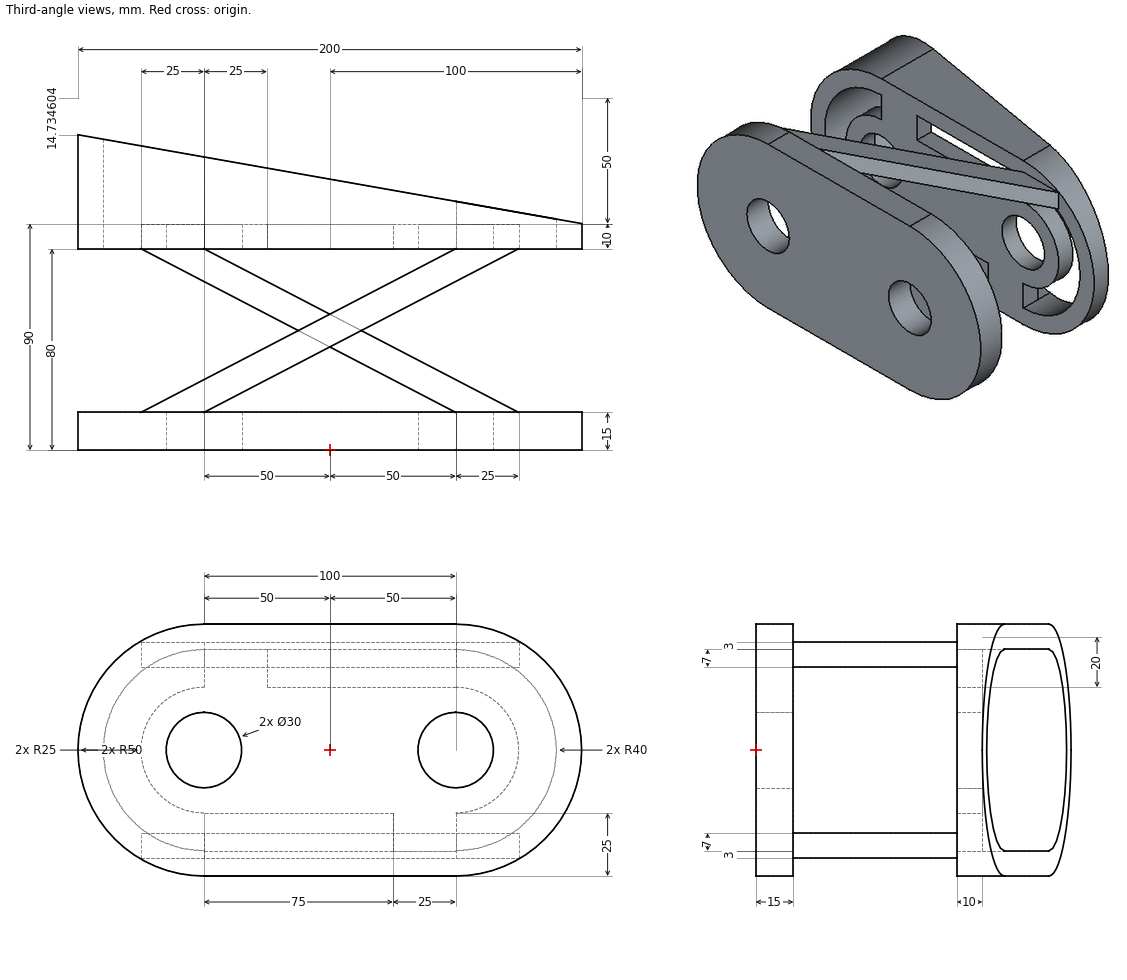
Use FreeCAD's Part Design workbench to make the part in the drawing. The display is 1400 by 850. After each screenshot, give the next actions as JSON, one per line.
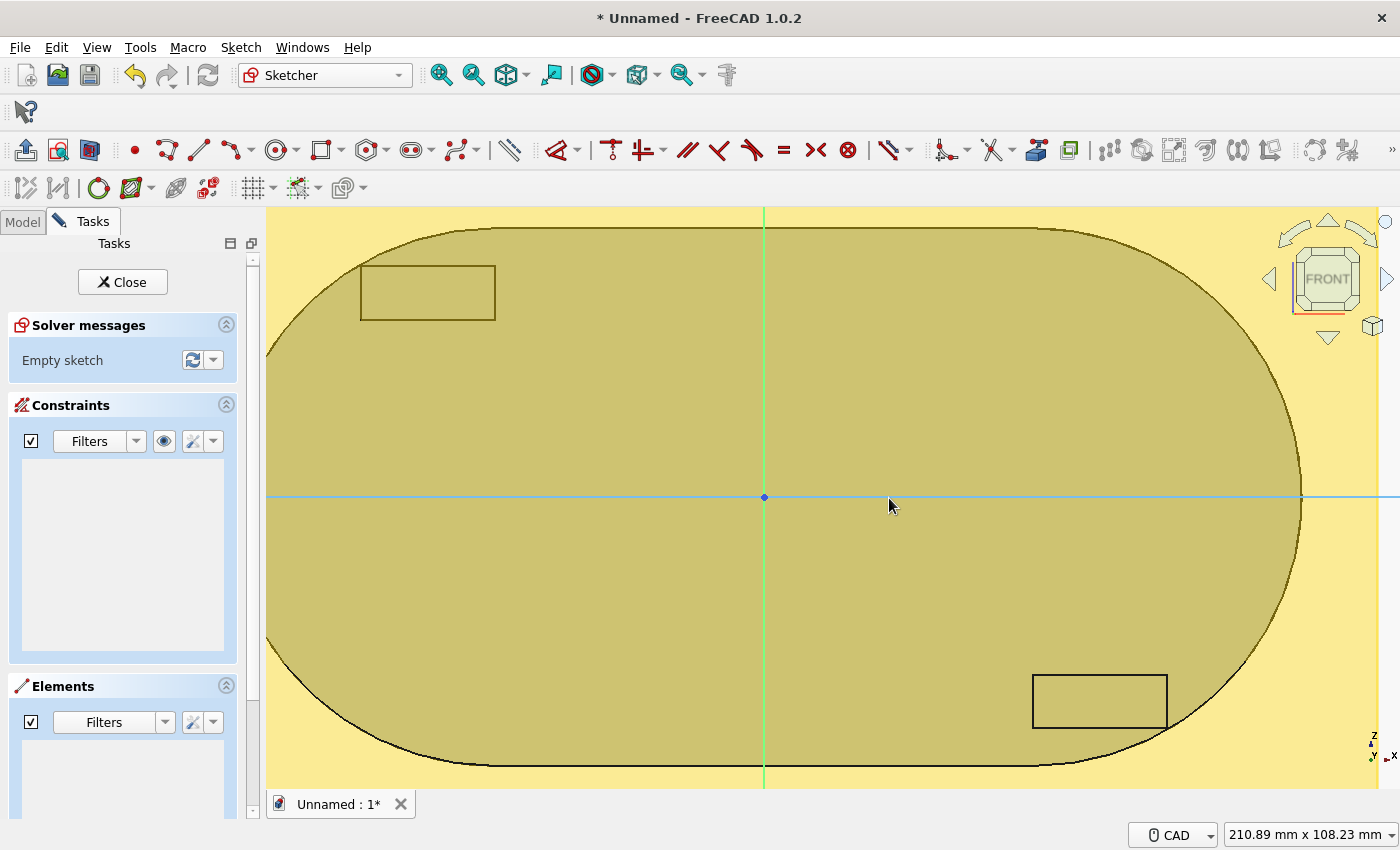
{"action": "left_click", "coordinate": [276, 150]}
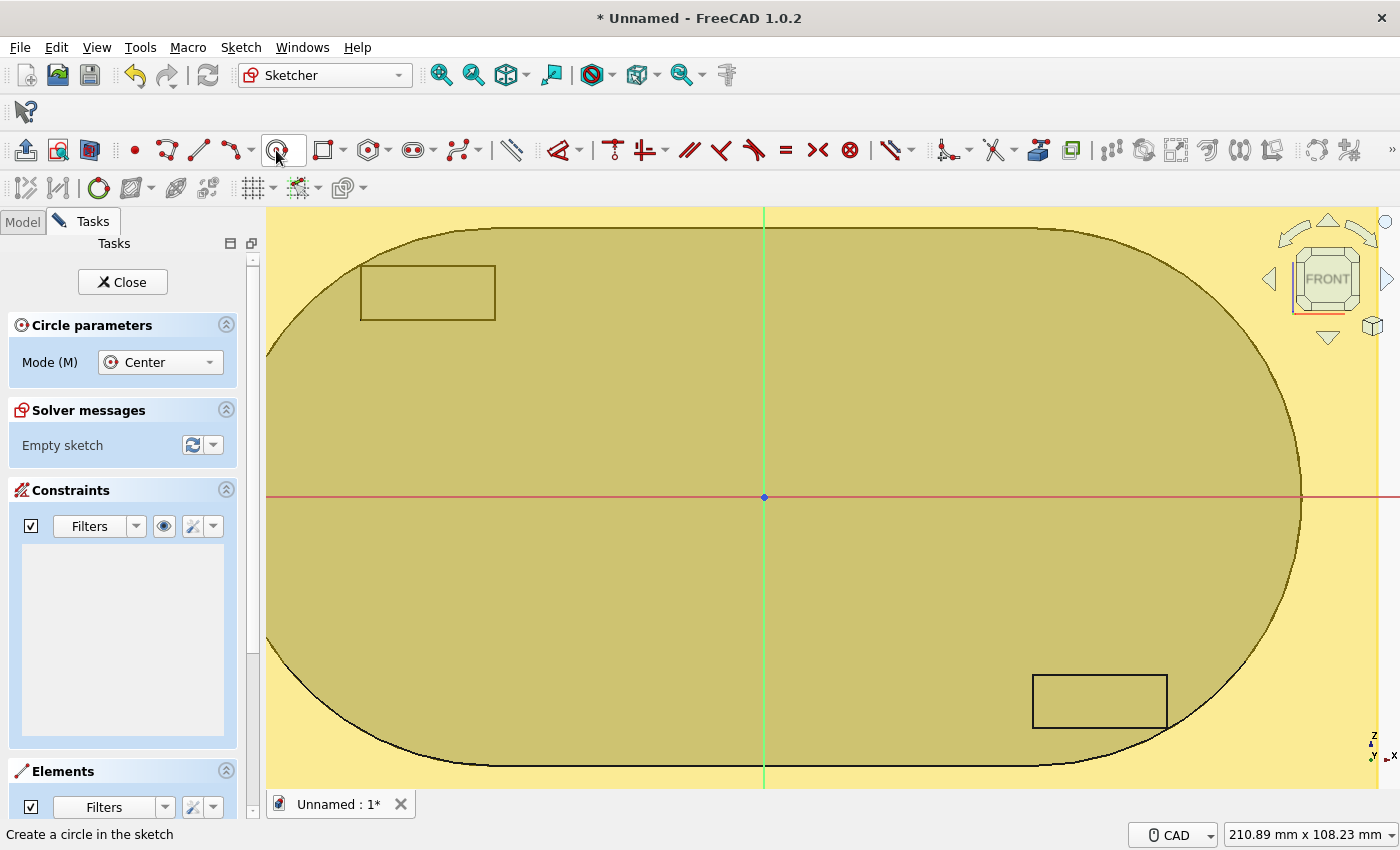
{"action": "left_click", "coordinate": [495, 497]}
{"action": "left_click", "coordinate": [552, 440]}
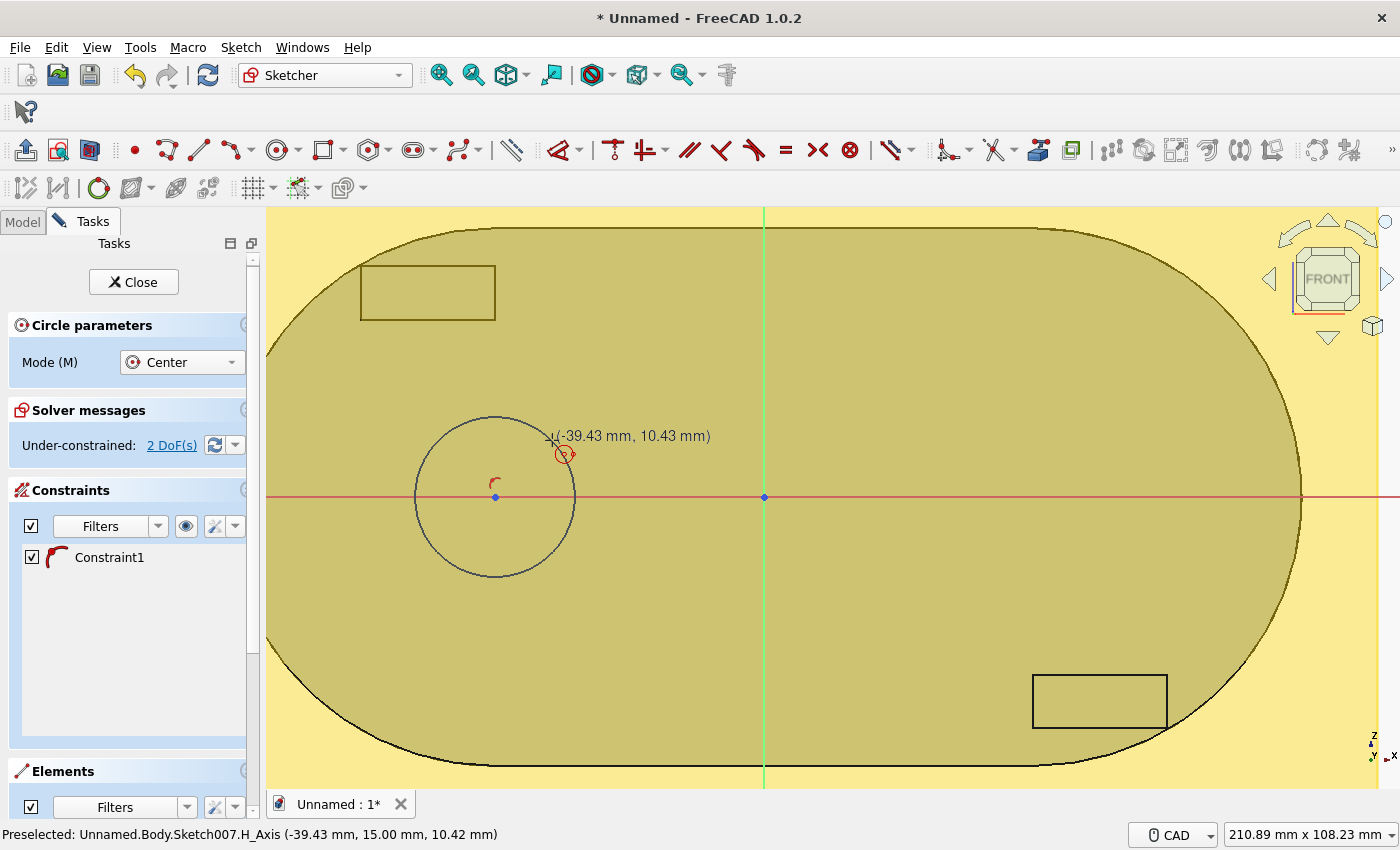
{"action": "left_click", "coordinate": [1033, 497]}
{"action": "left_click", "coordinate": [1090, 440]}
{"action": "key", "text": "Escape"}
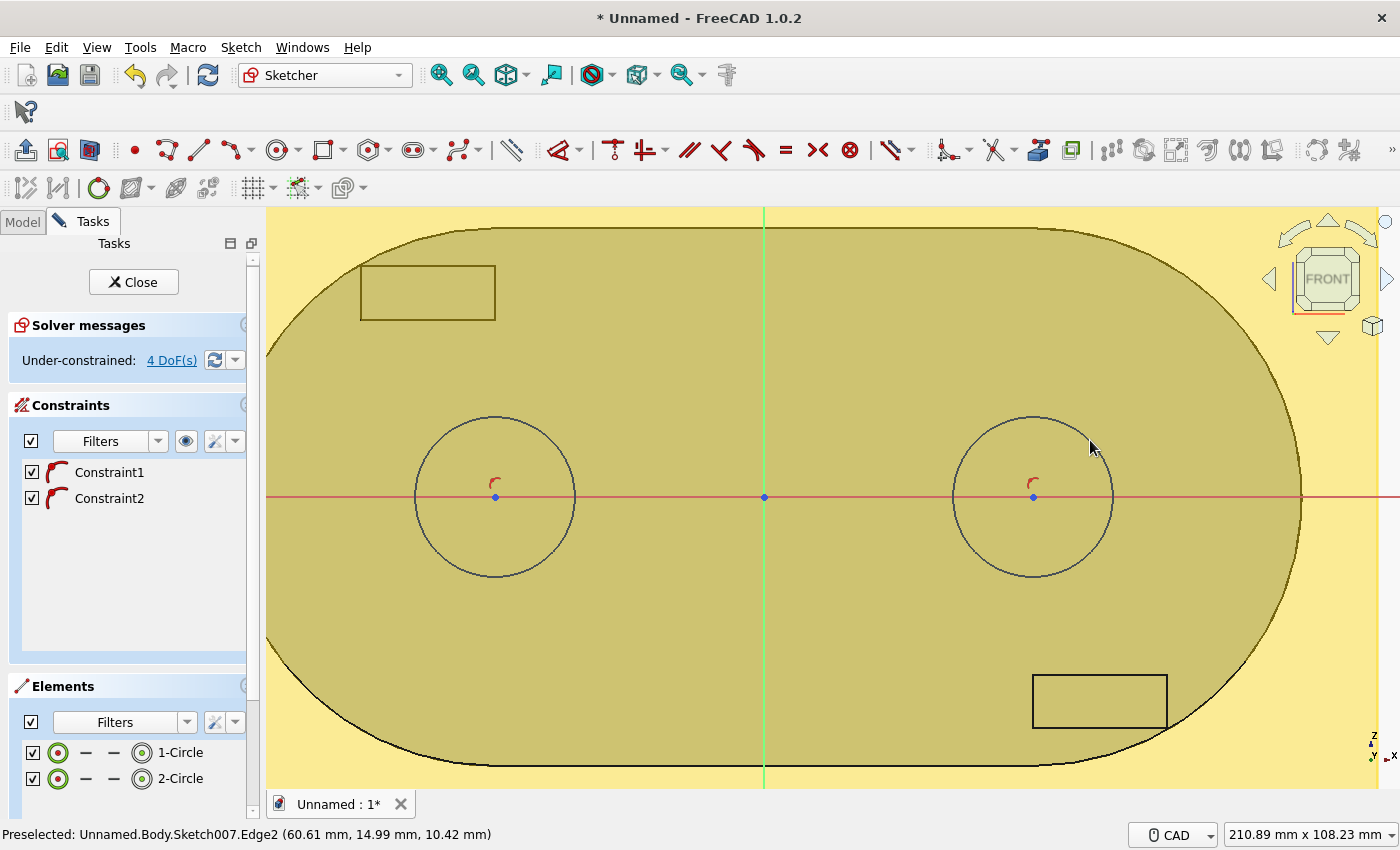
{"action": "left_click", "coordinate": [551, 440]}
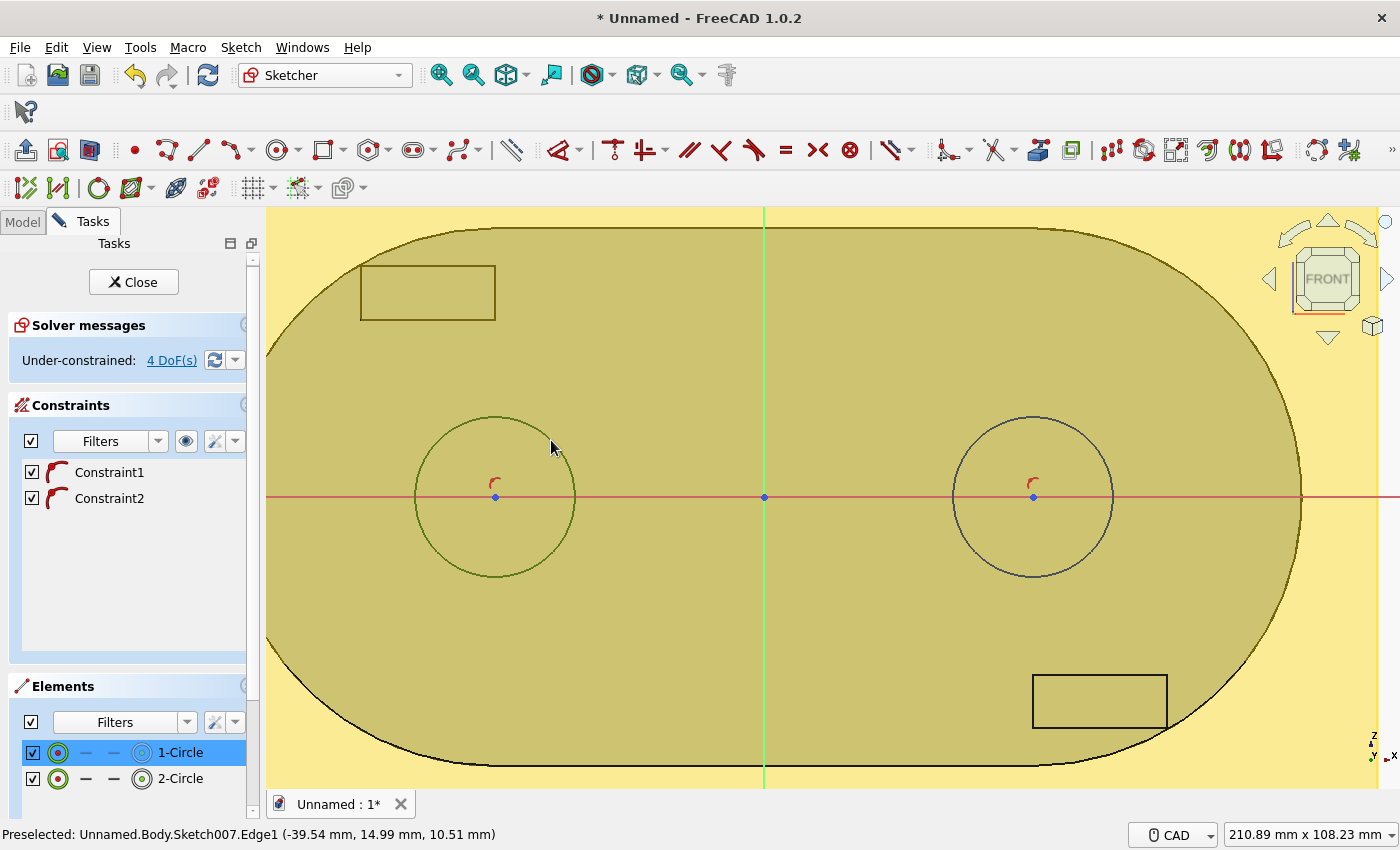
{"action": "left_click", "coordinate": [1089, 440]}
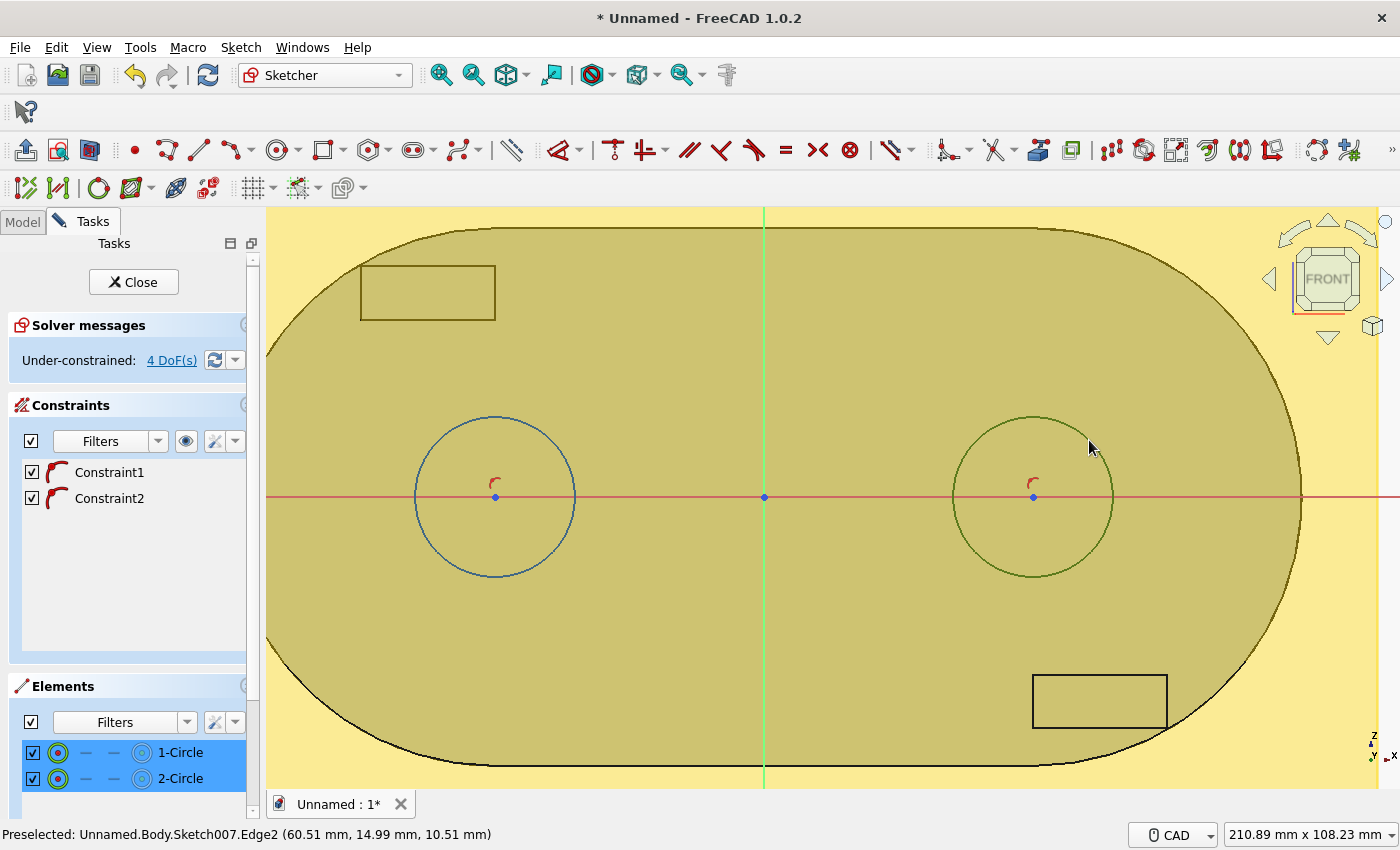
{"action": "left_click", "coordinate": [786, 150]}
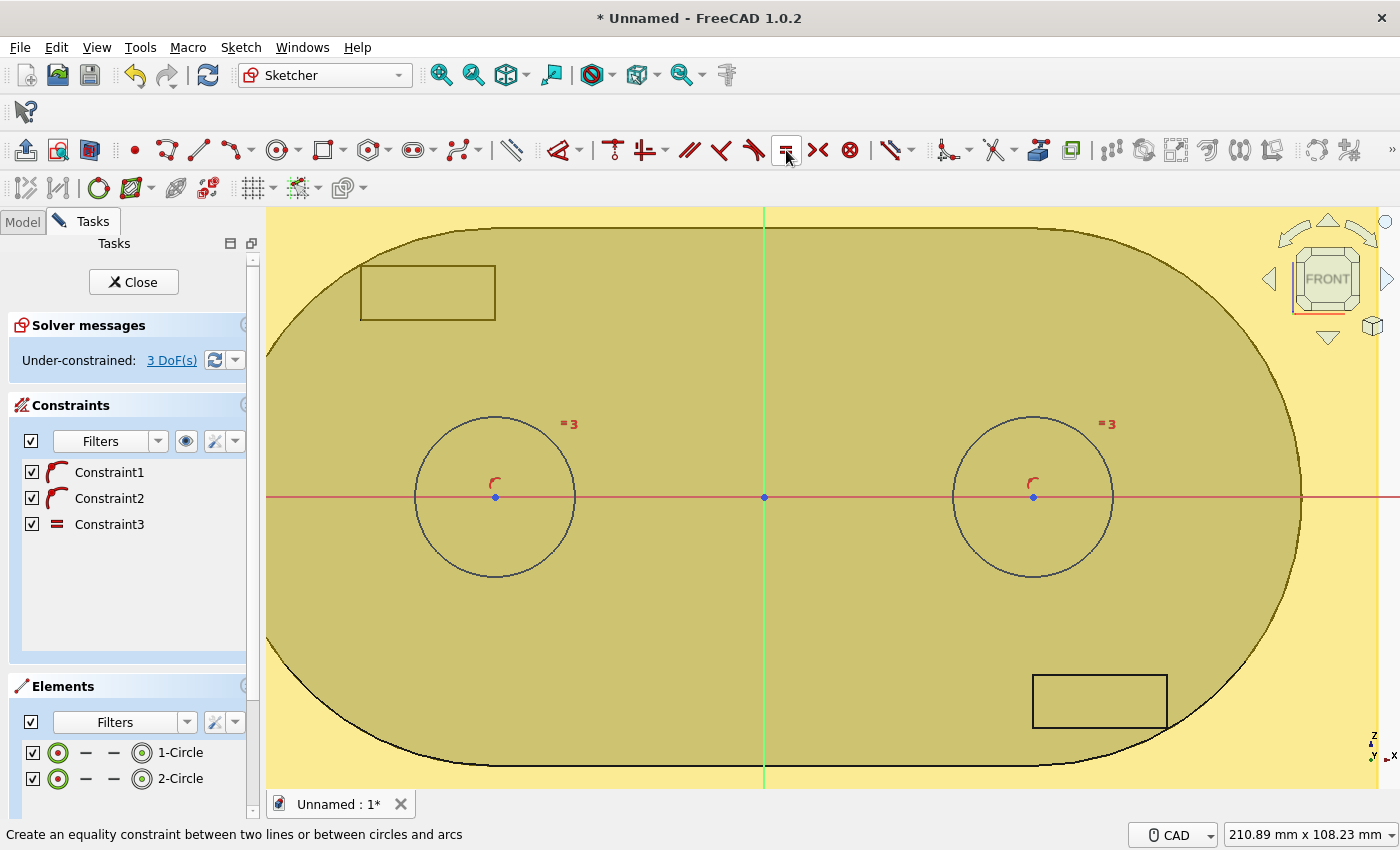
{"action": "key", "text": "d"}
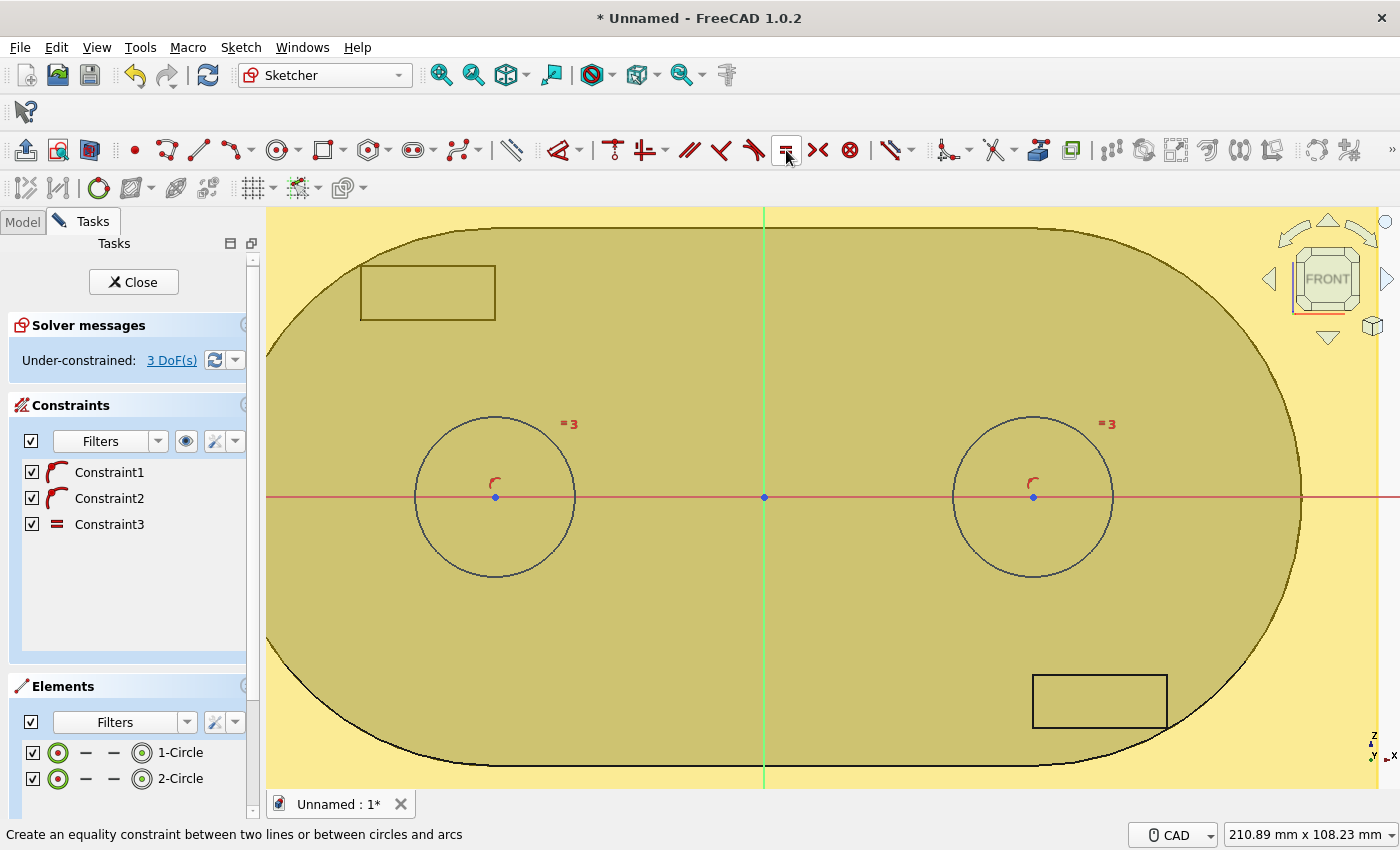
{"action": "left_click", "coordinate": [551, 440]}
{"action": "left_click", "coordinate": [573, 417]}